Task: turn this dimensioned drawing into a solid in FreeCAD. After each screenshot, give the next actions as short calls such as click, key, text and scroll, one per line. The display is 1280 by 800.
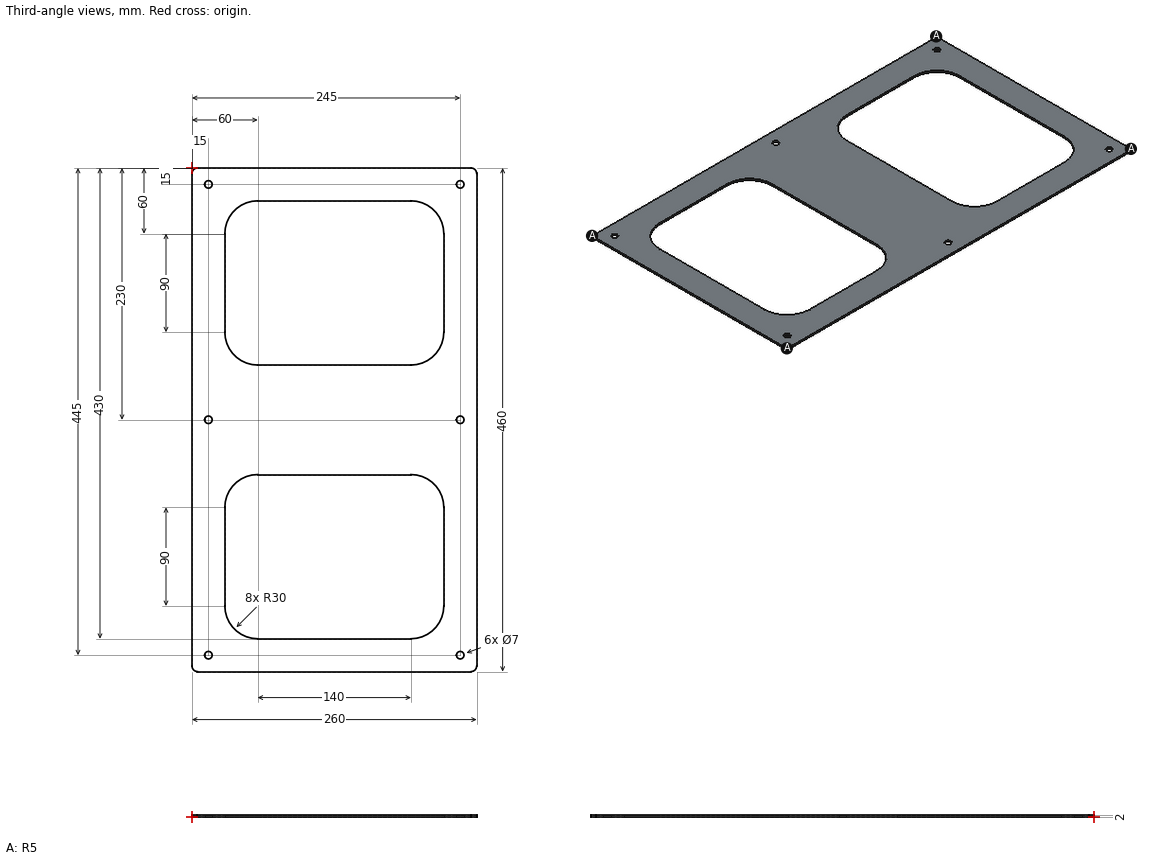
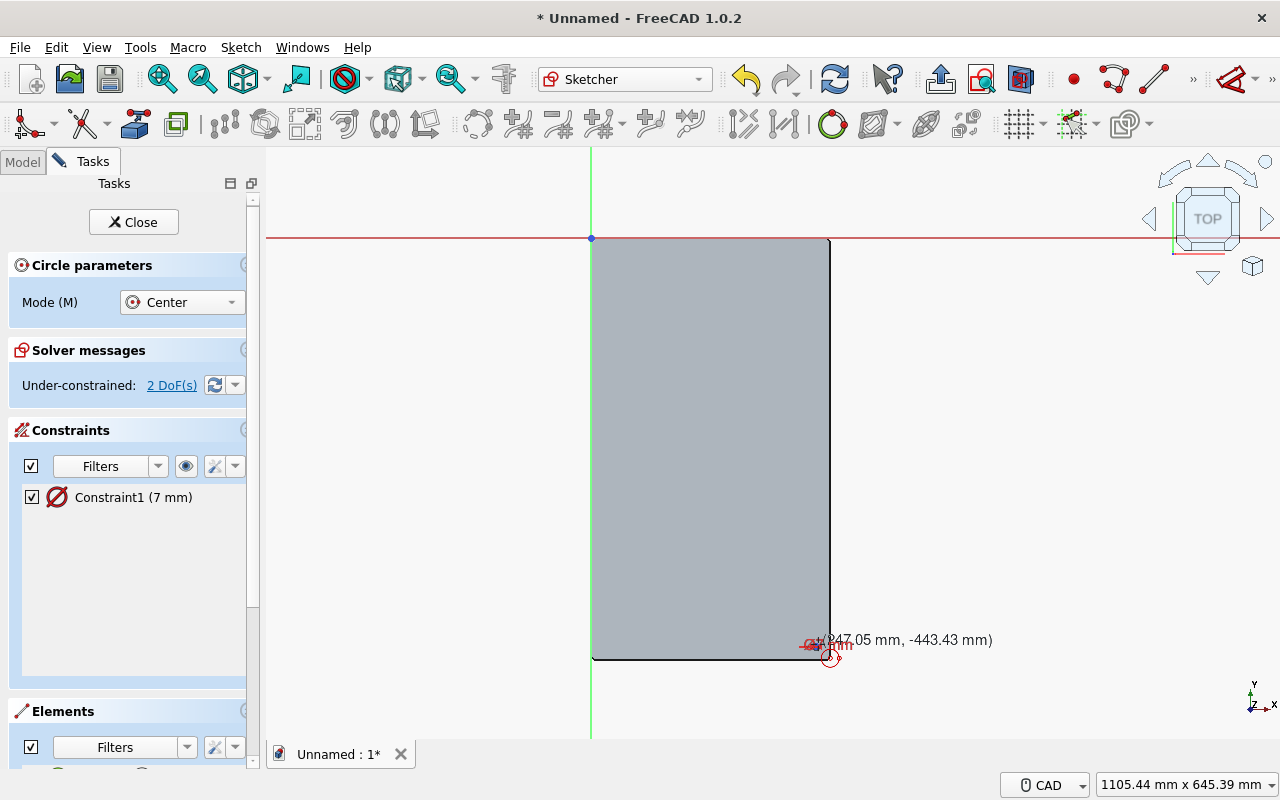
scroll(605, 646, up, 10)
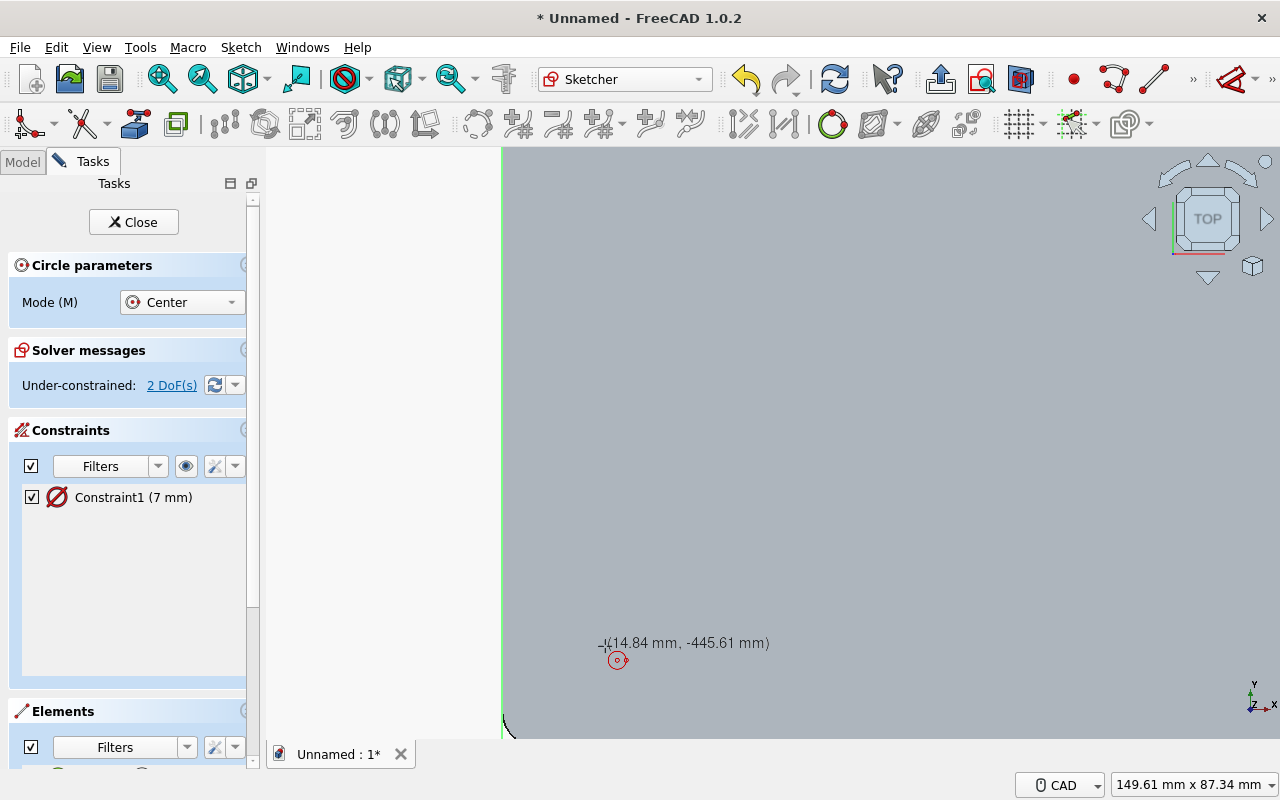
scroll(604, 646, down, 10)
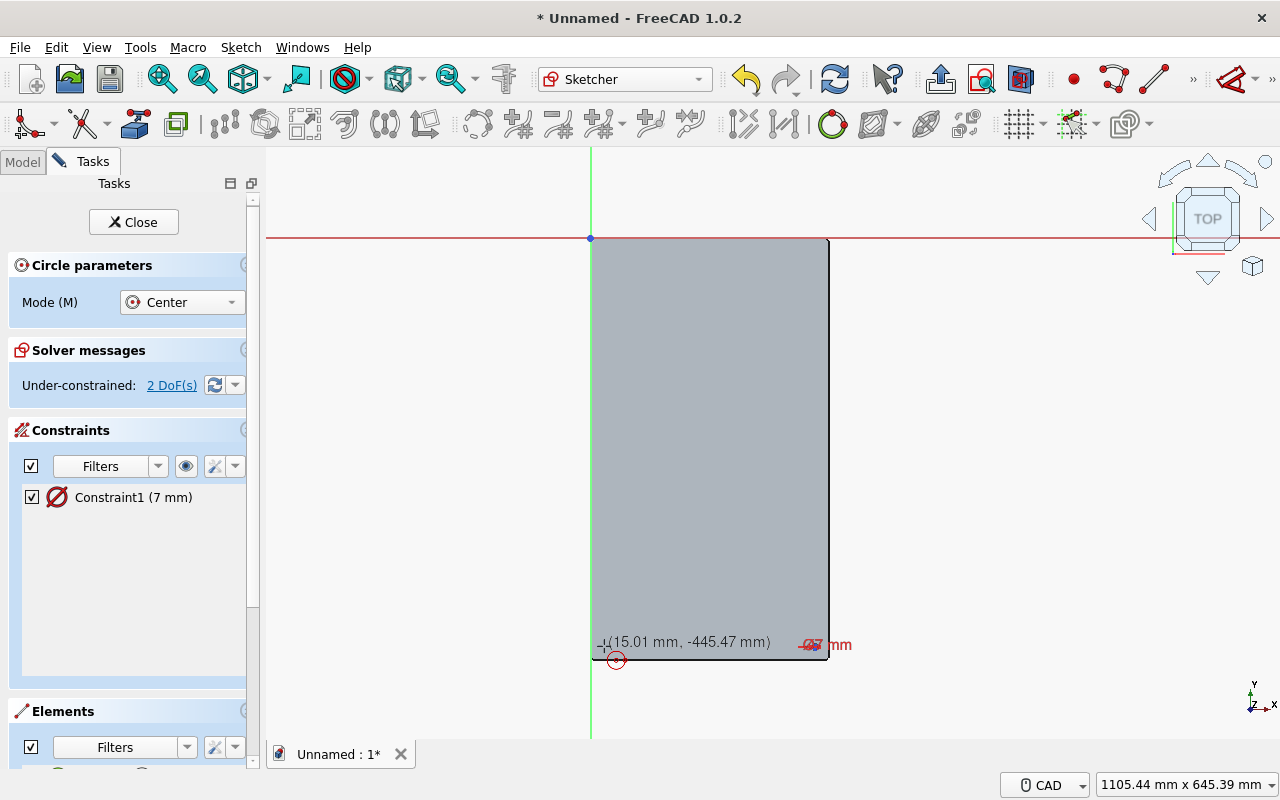
click(604, 646)
move(607, 644)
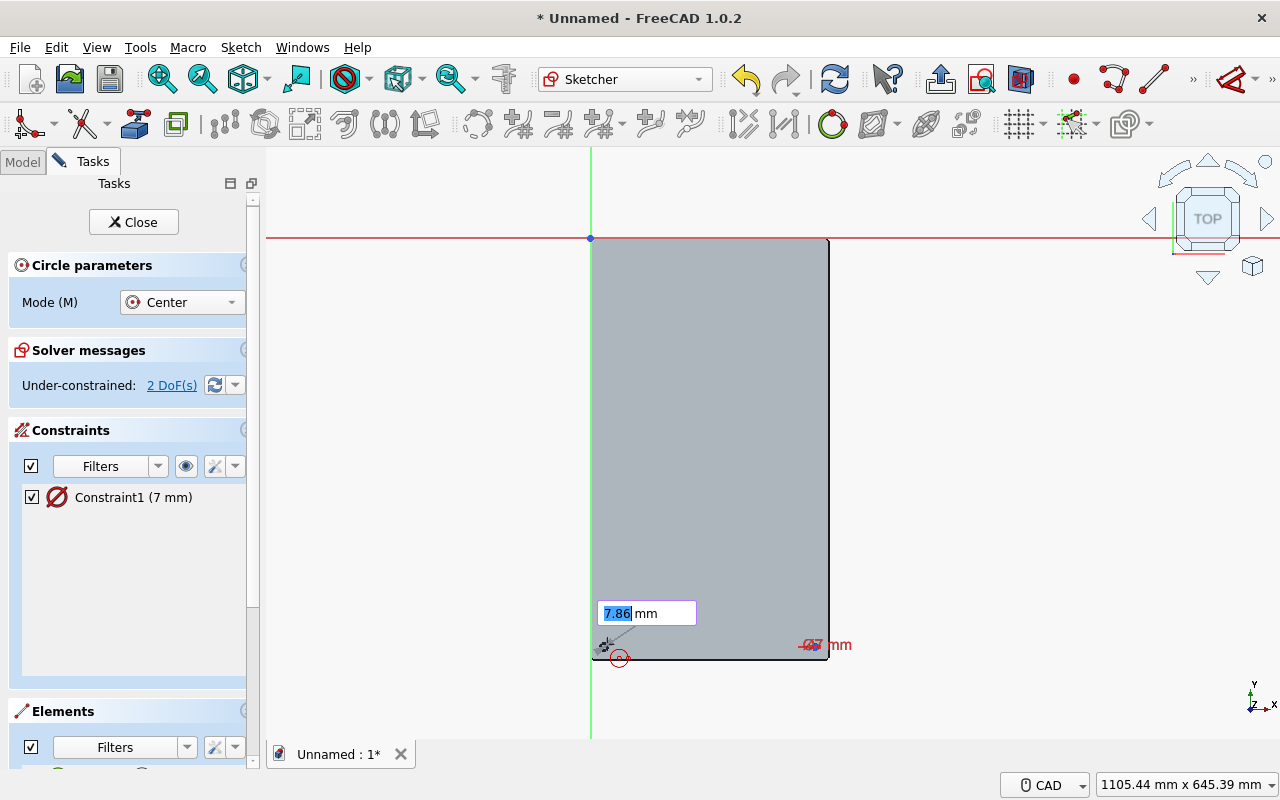
text(7)
key(Return)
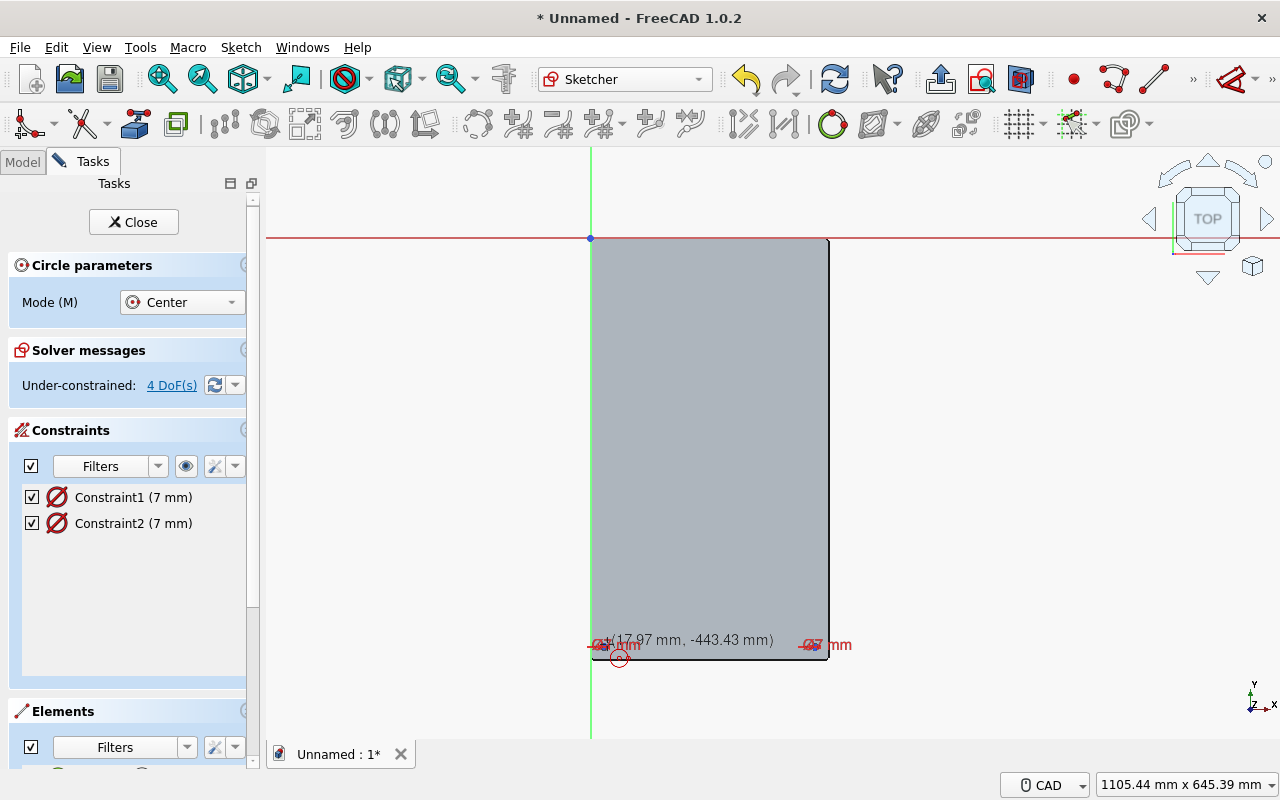
scroll(815, 252, up, 10)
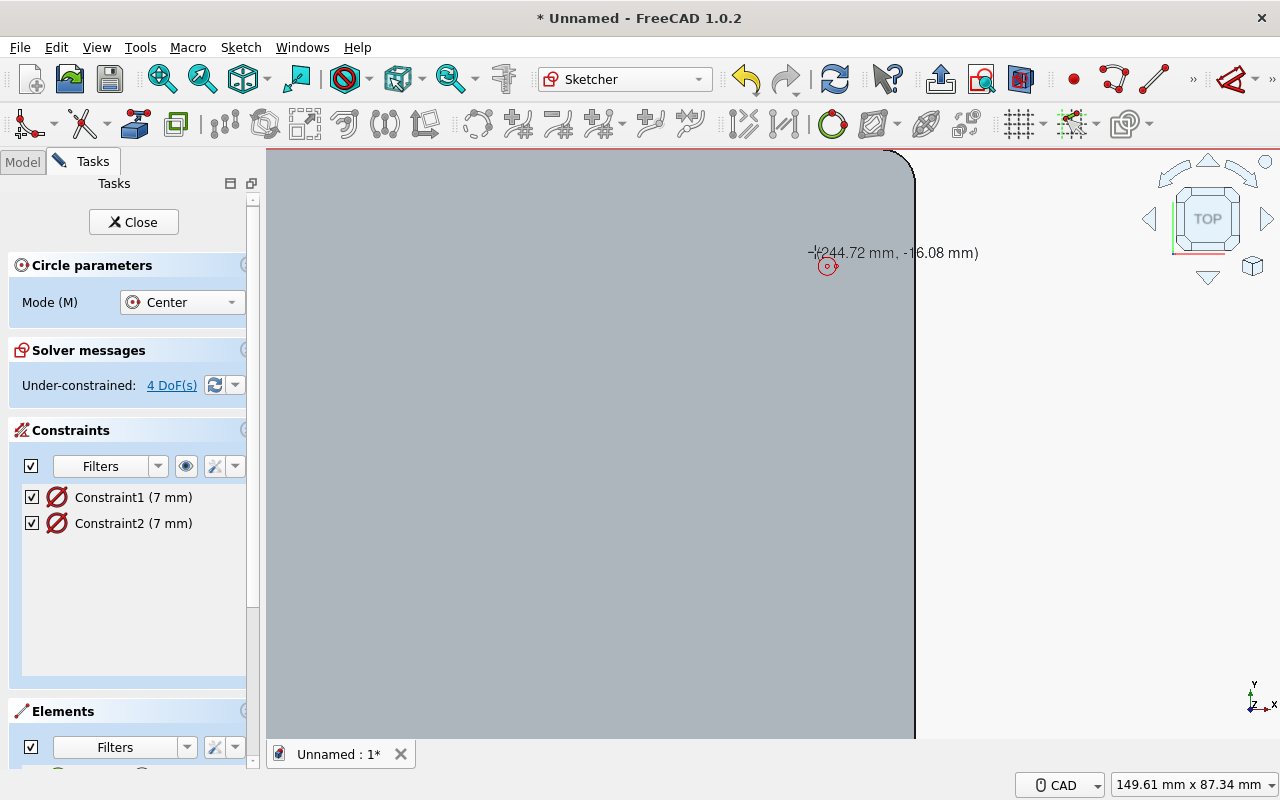
scroll(816, 251, down, 10)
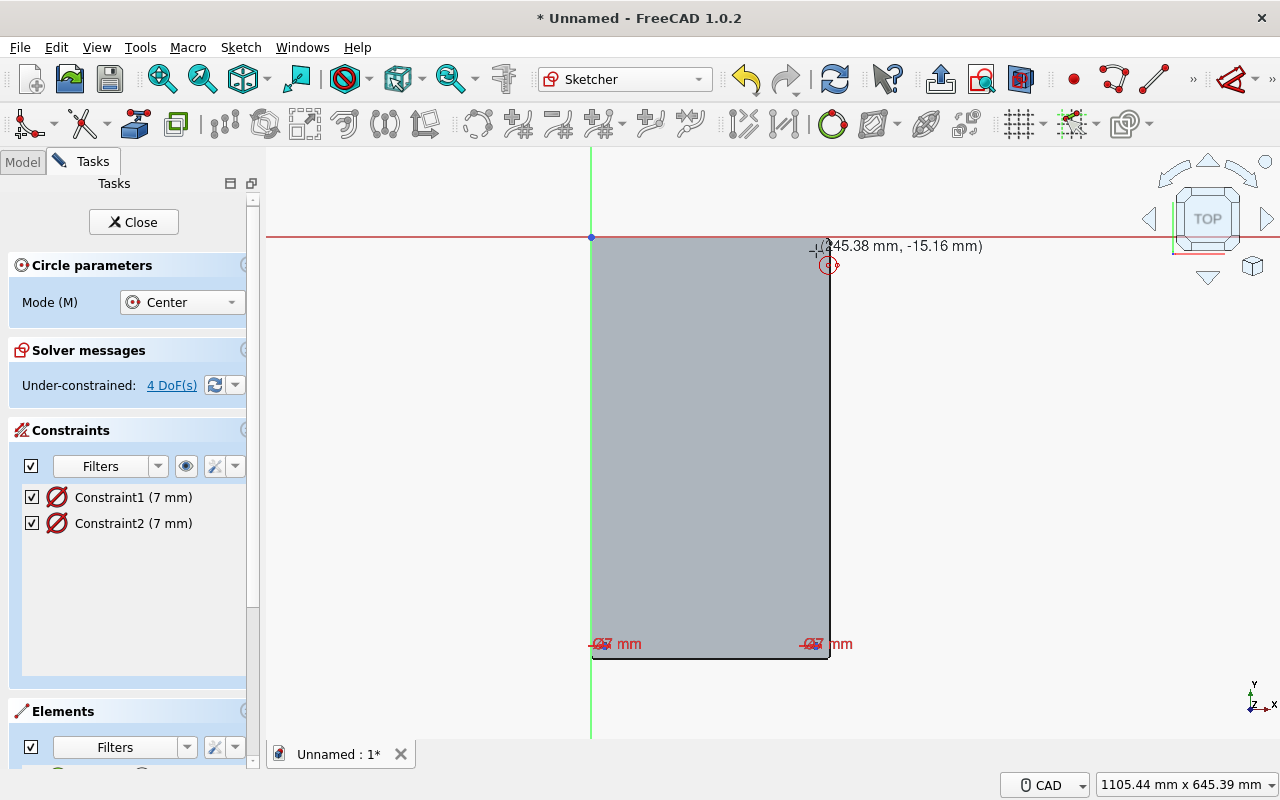
click(816, 251)
move(818, 253)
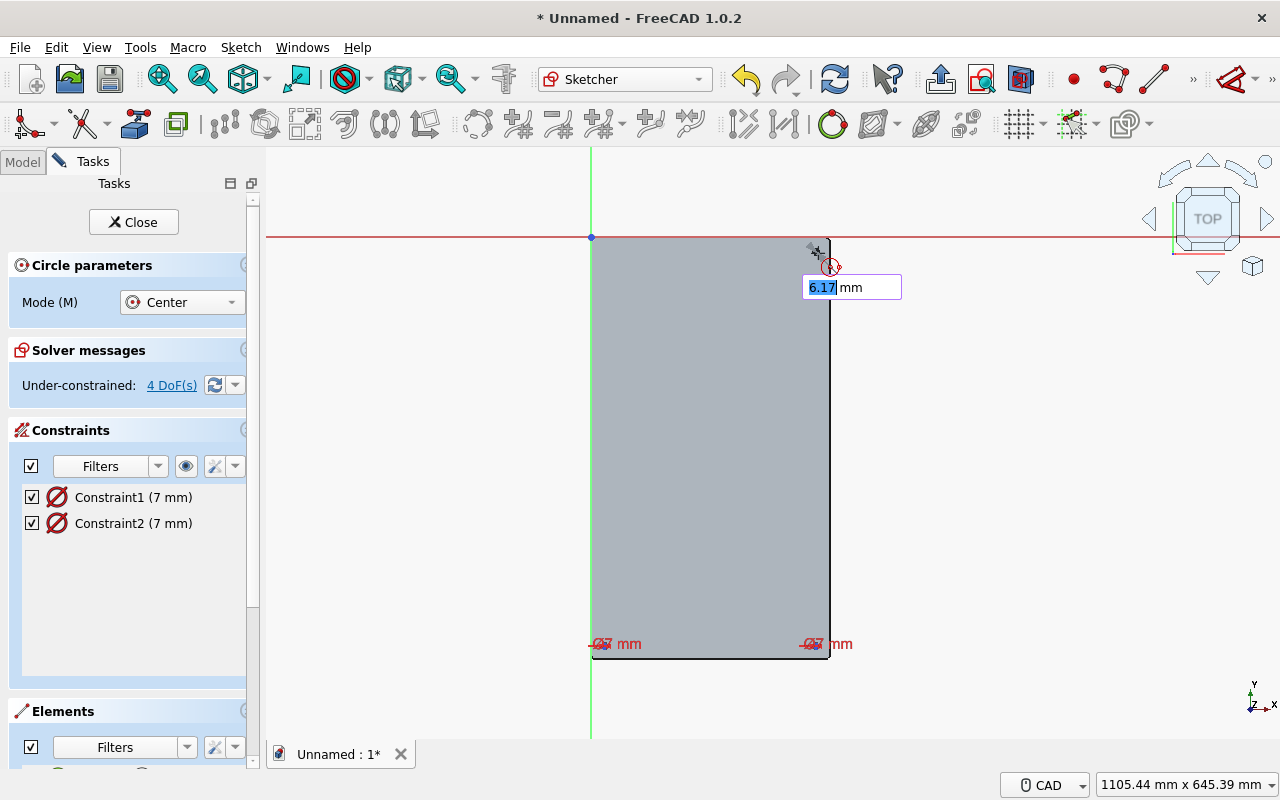
text(7)
key(Return)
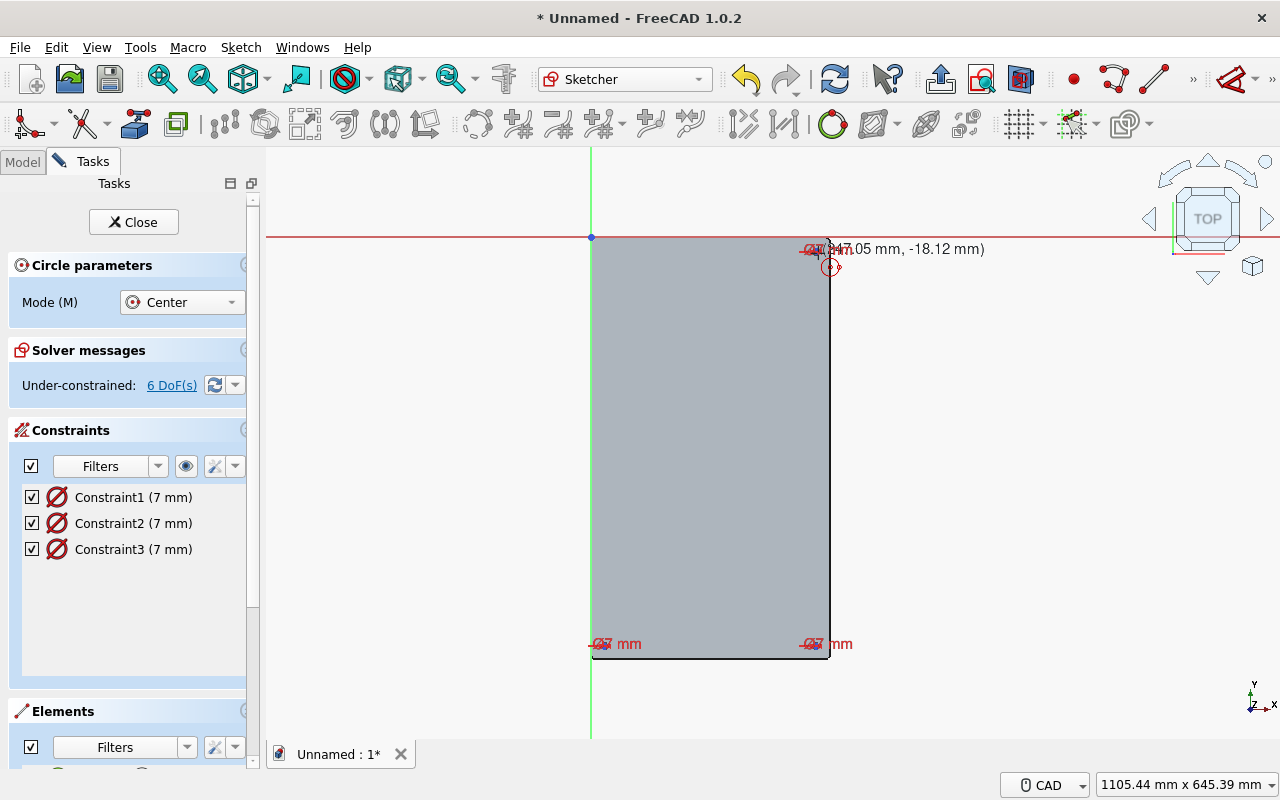
scroll(605, 251, up, 10)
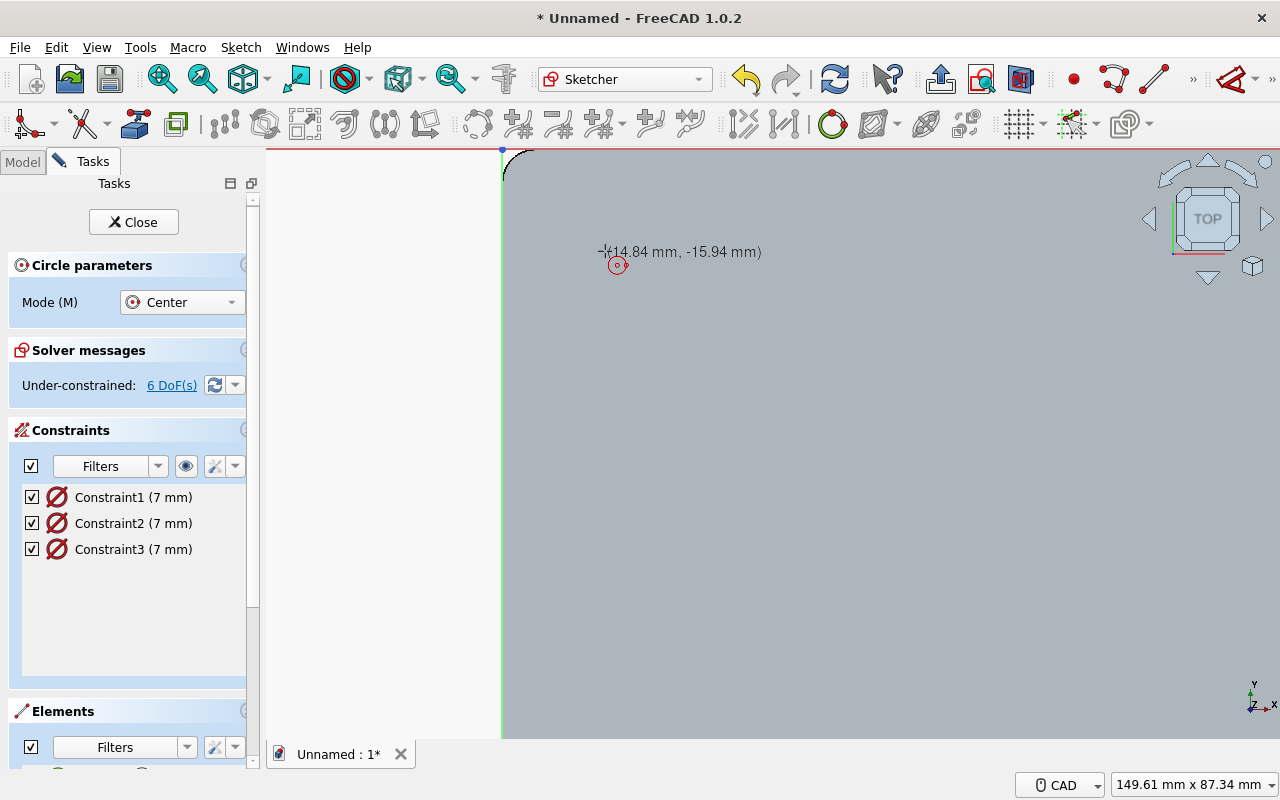
scroll(604, 251, down, 10)